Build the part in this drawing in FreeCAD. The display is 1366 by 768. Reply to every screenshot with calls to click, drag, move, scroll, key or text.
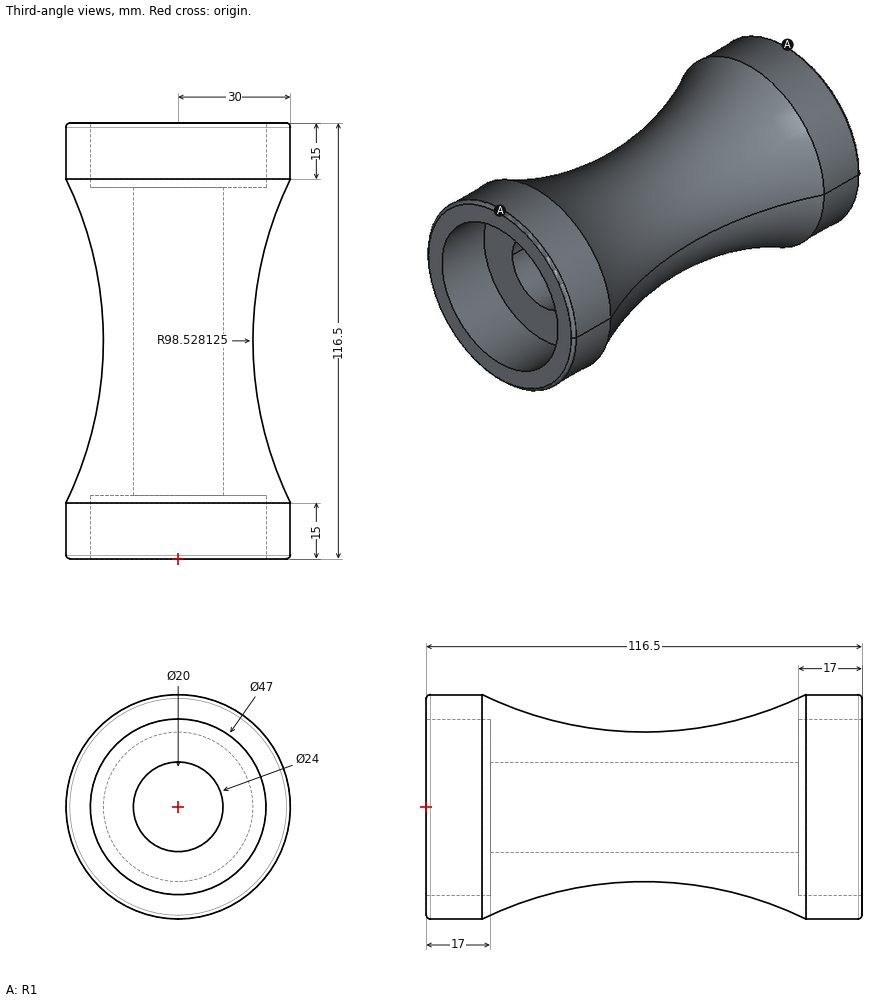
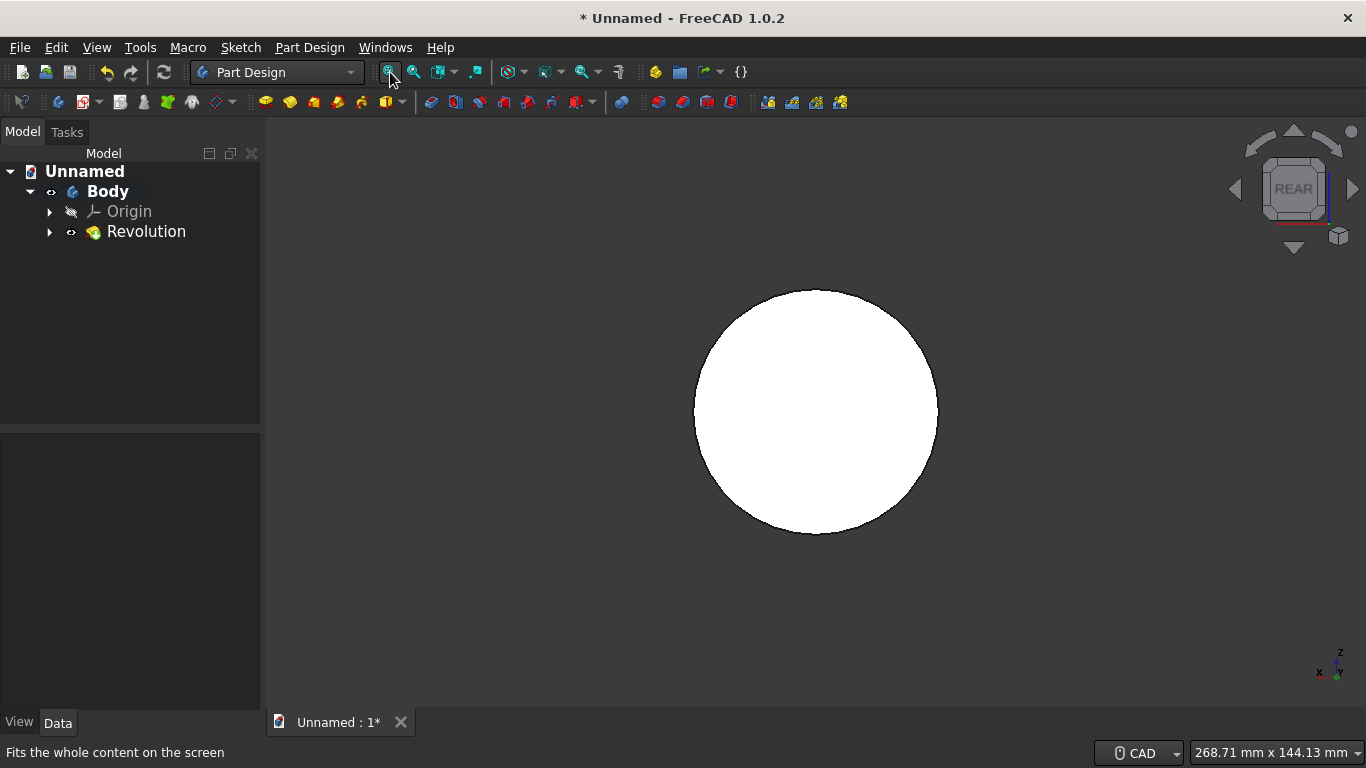
click(816, 411)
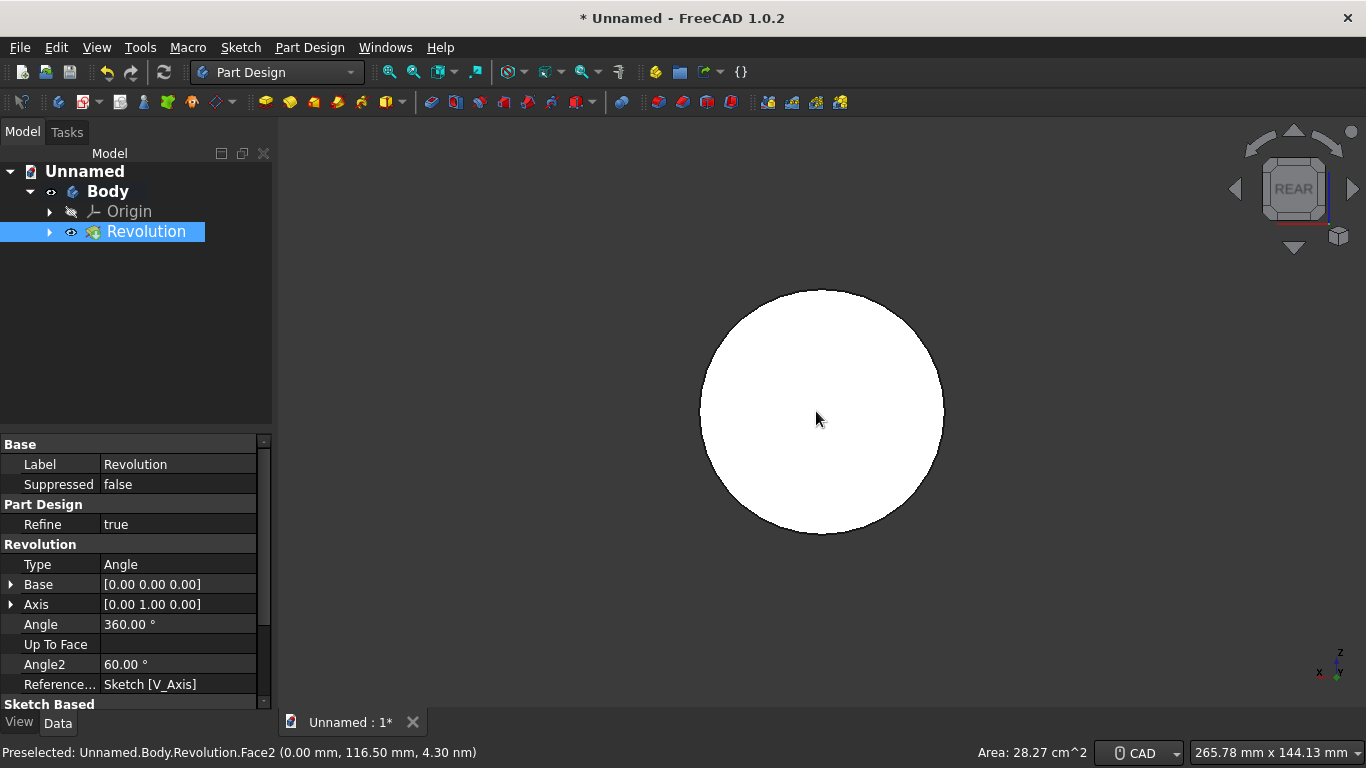
click(84, 102)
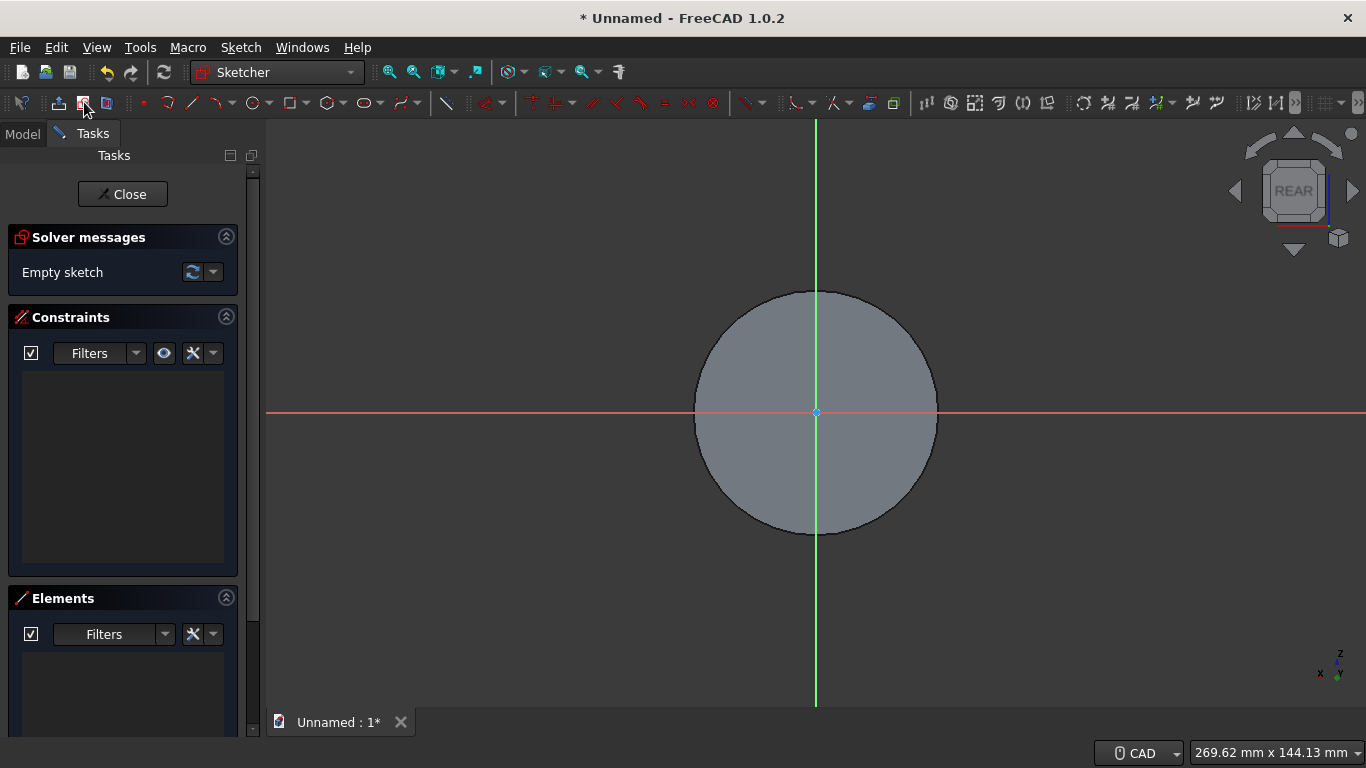
scroll(838, 413, up, 7)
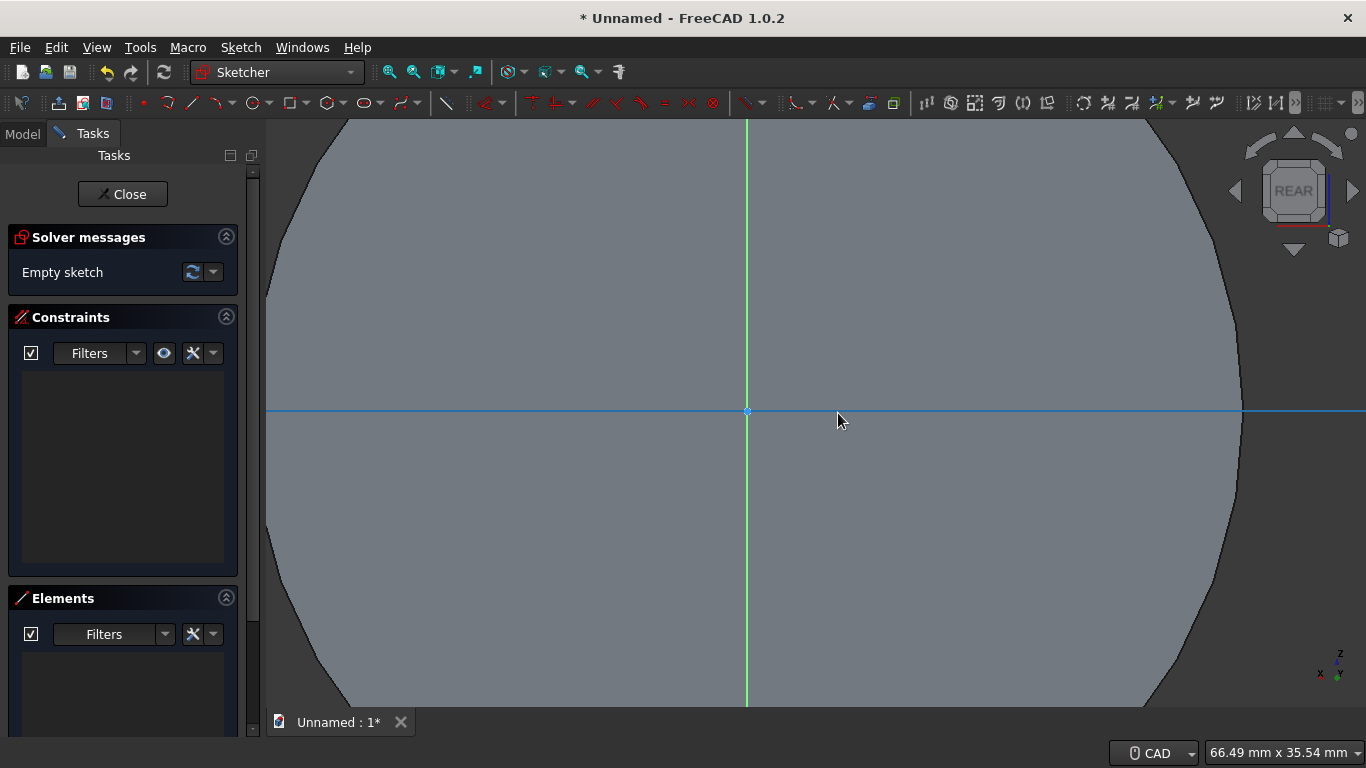
click(254, 104)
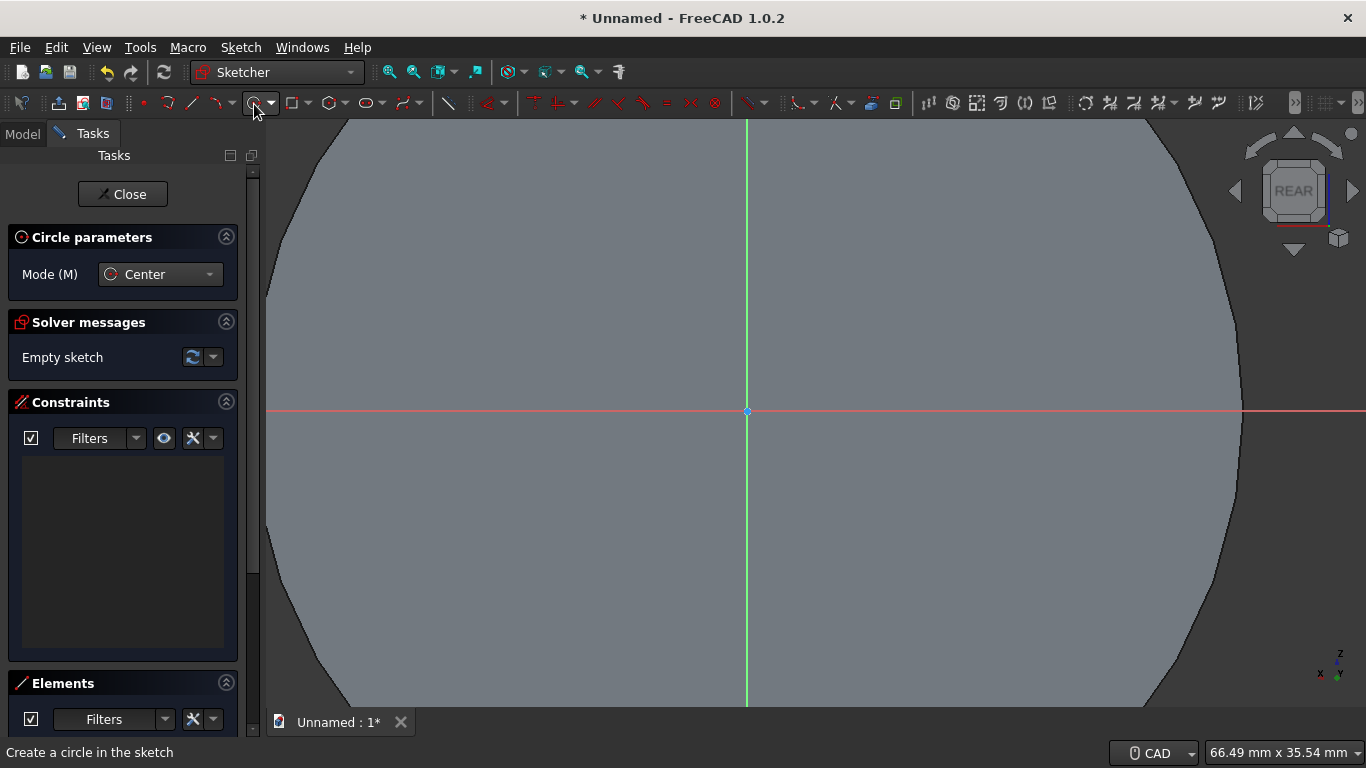
click(747, 411)
click(888, 271)
key(Escape)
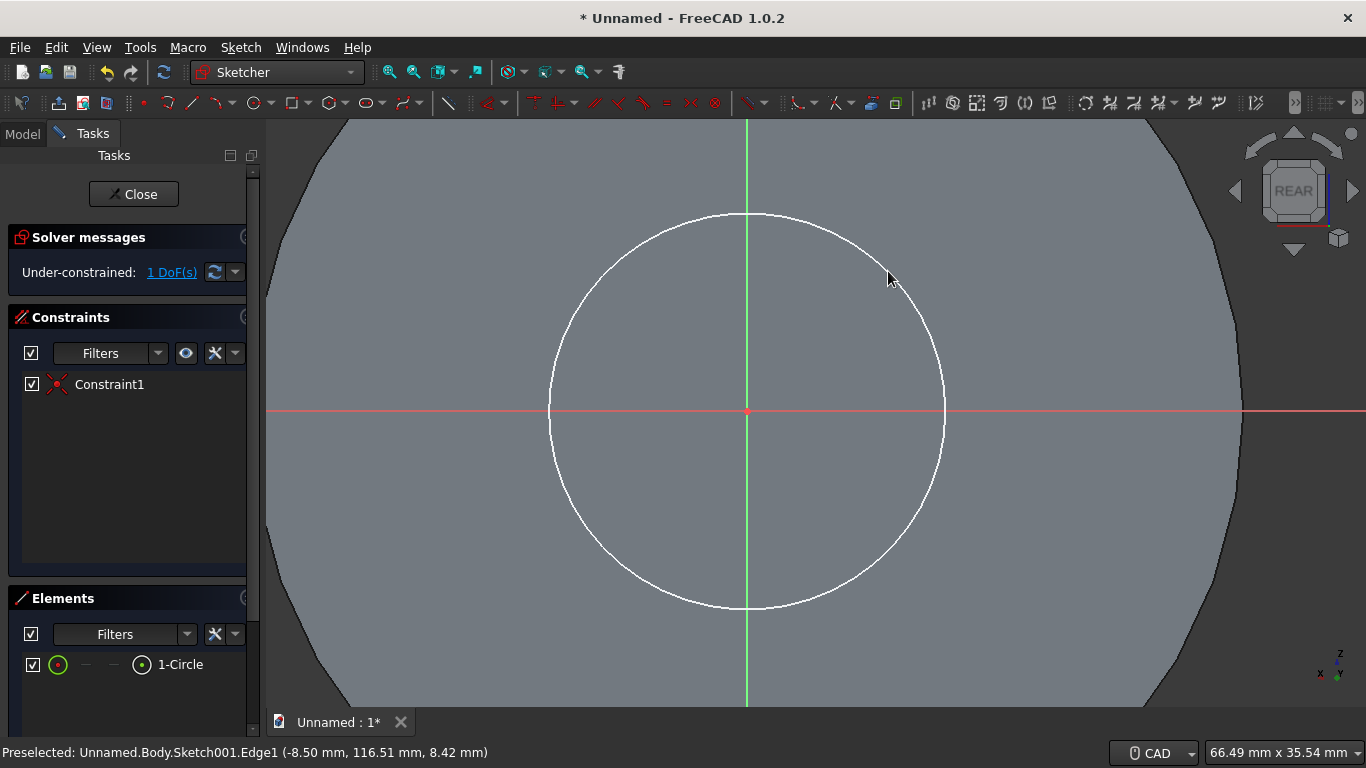
click(488, 104)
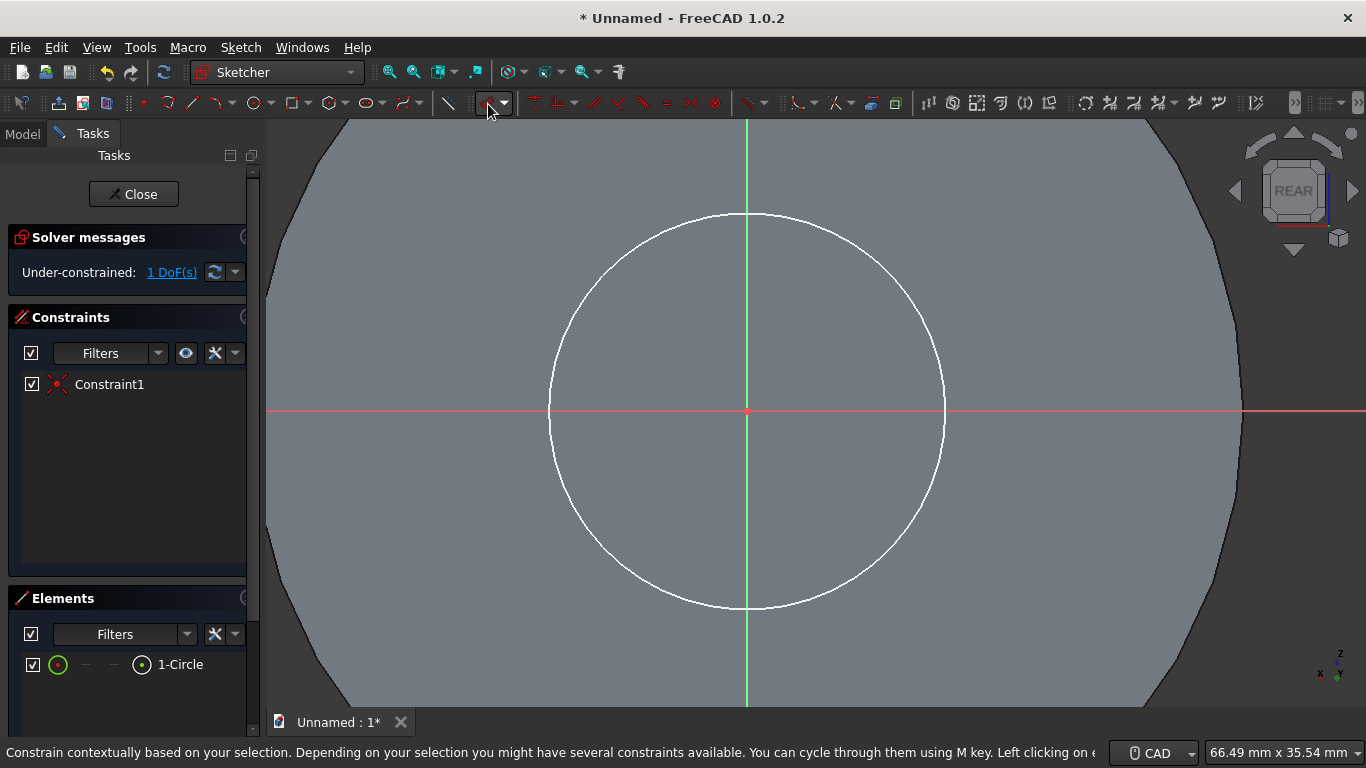
click(887, 271)
click(910, 248)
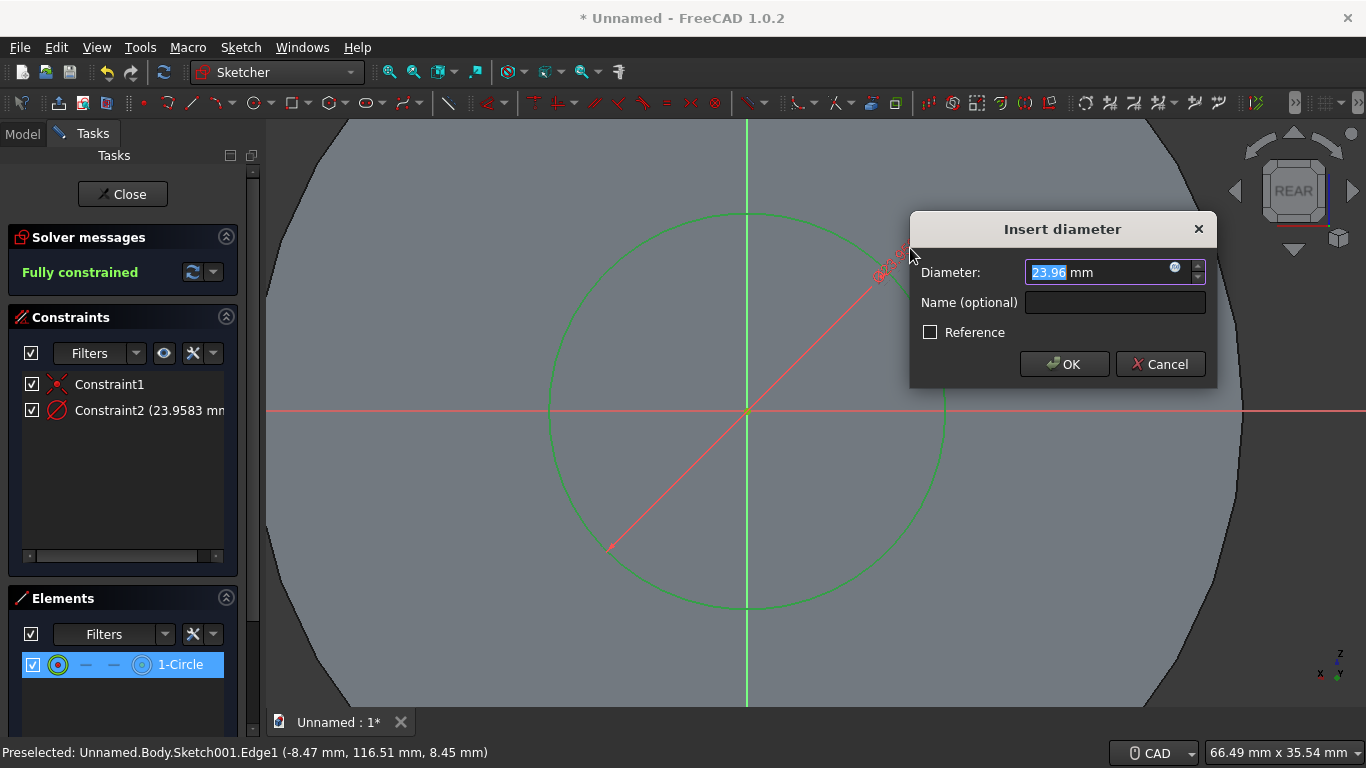
text(24)
key(Return)
key(Escape)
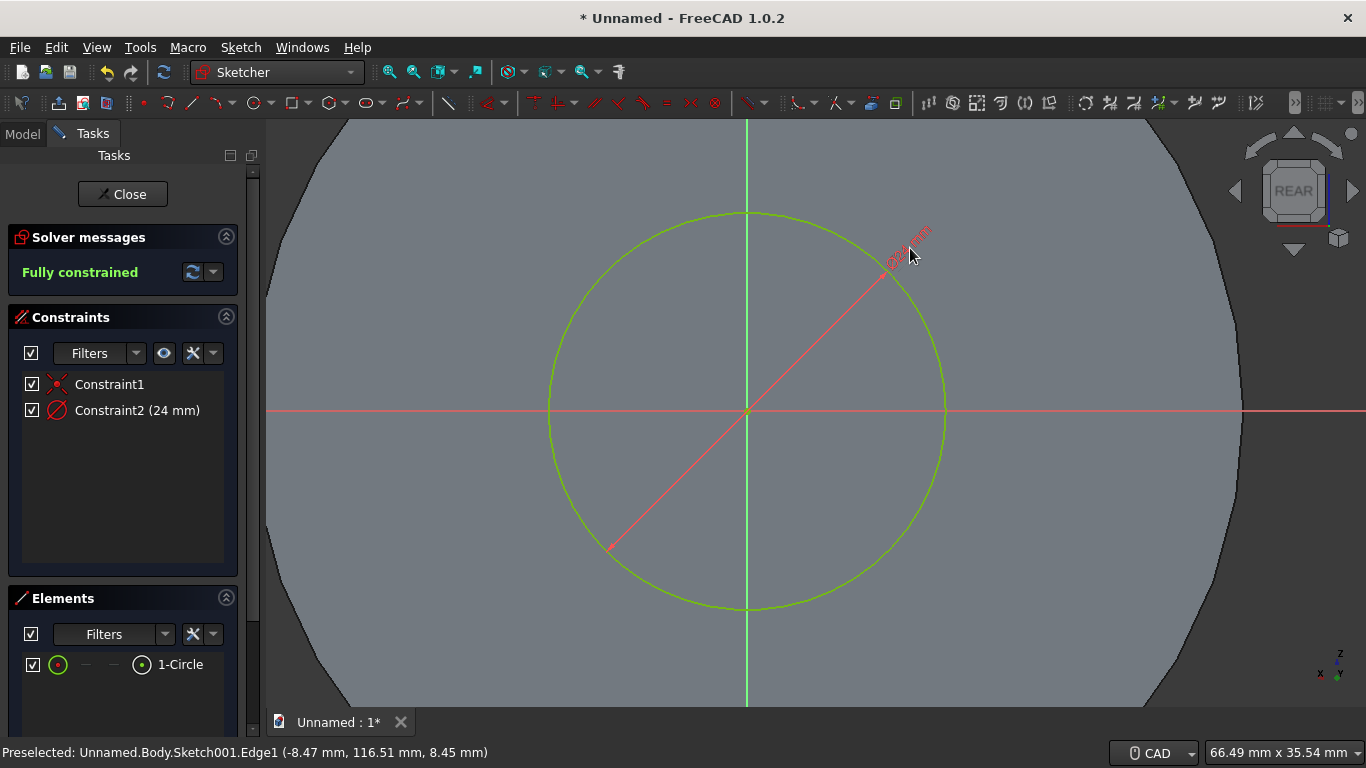
click(123, 194)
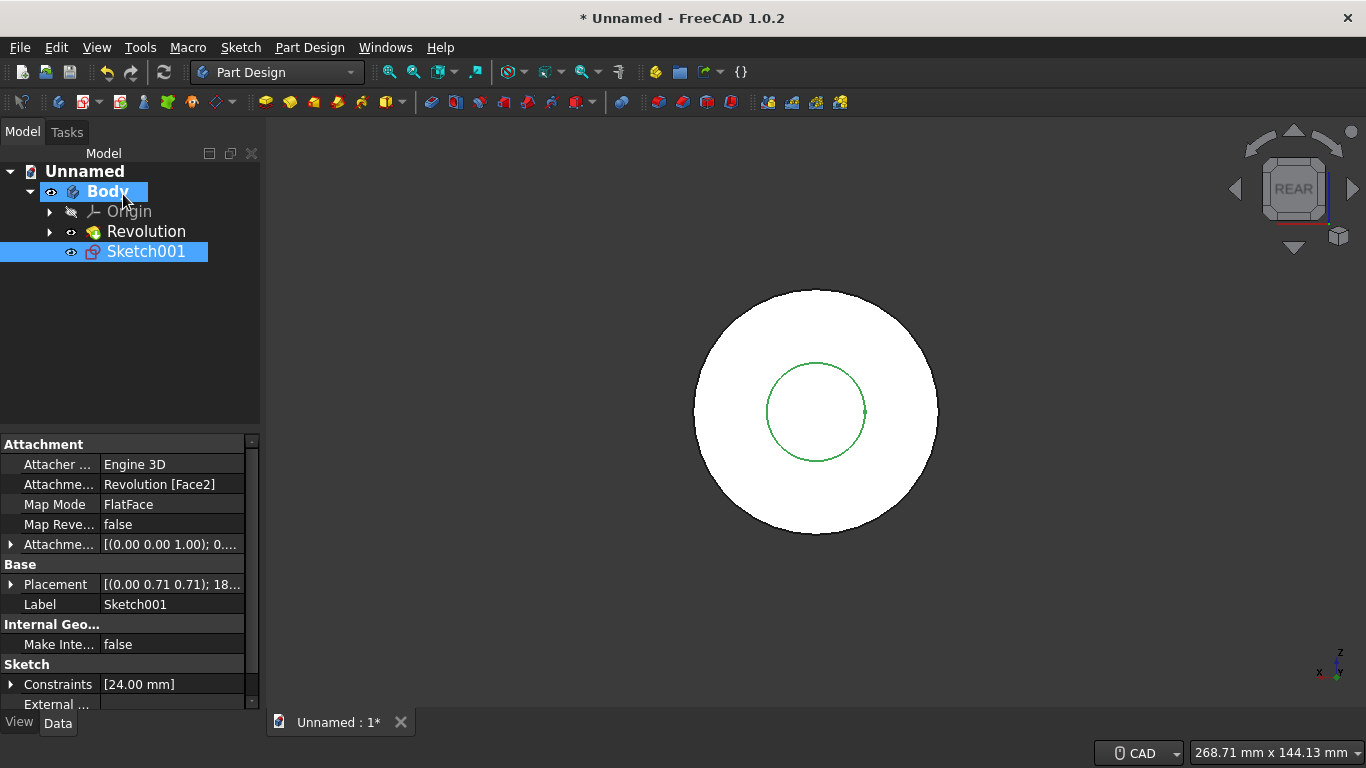
click(432, 102)